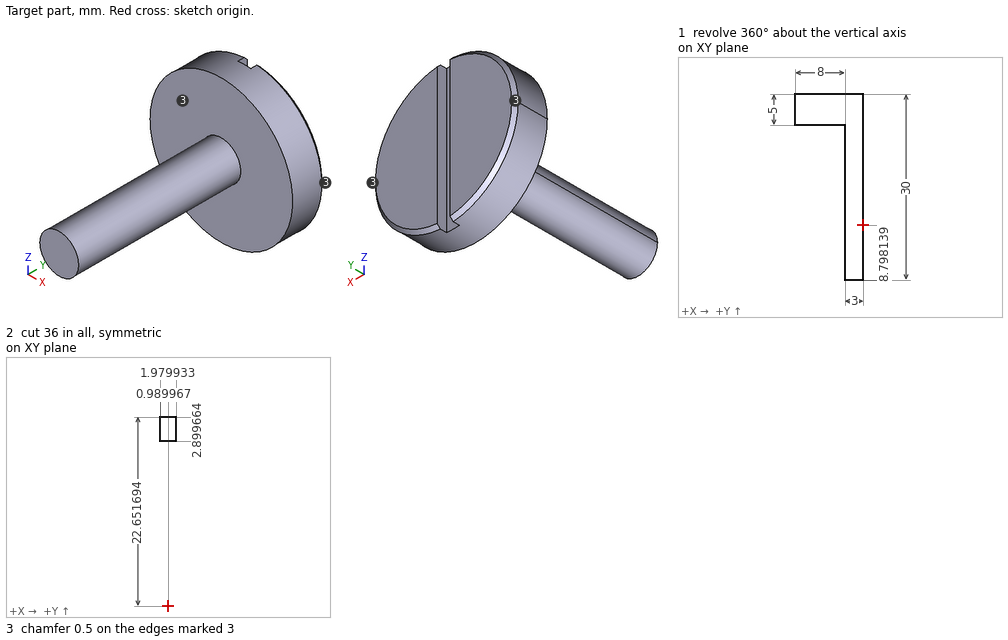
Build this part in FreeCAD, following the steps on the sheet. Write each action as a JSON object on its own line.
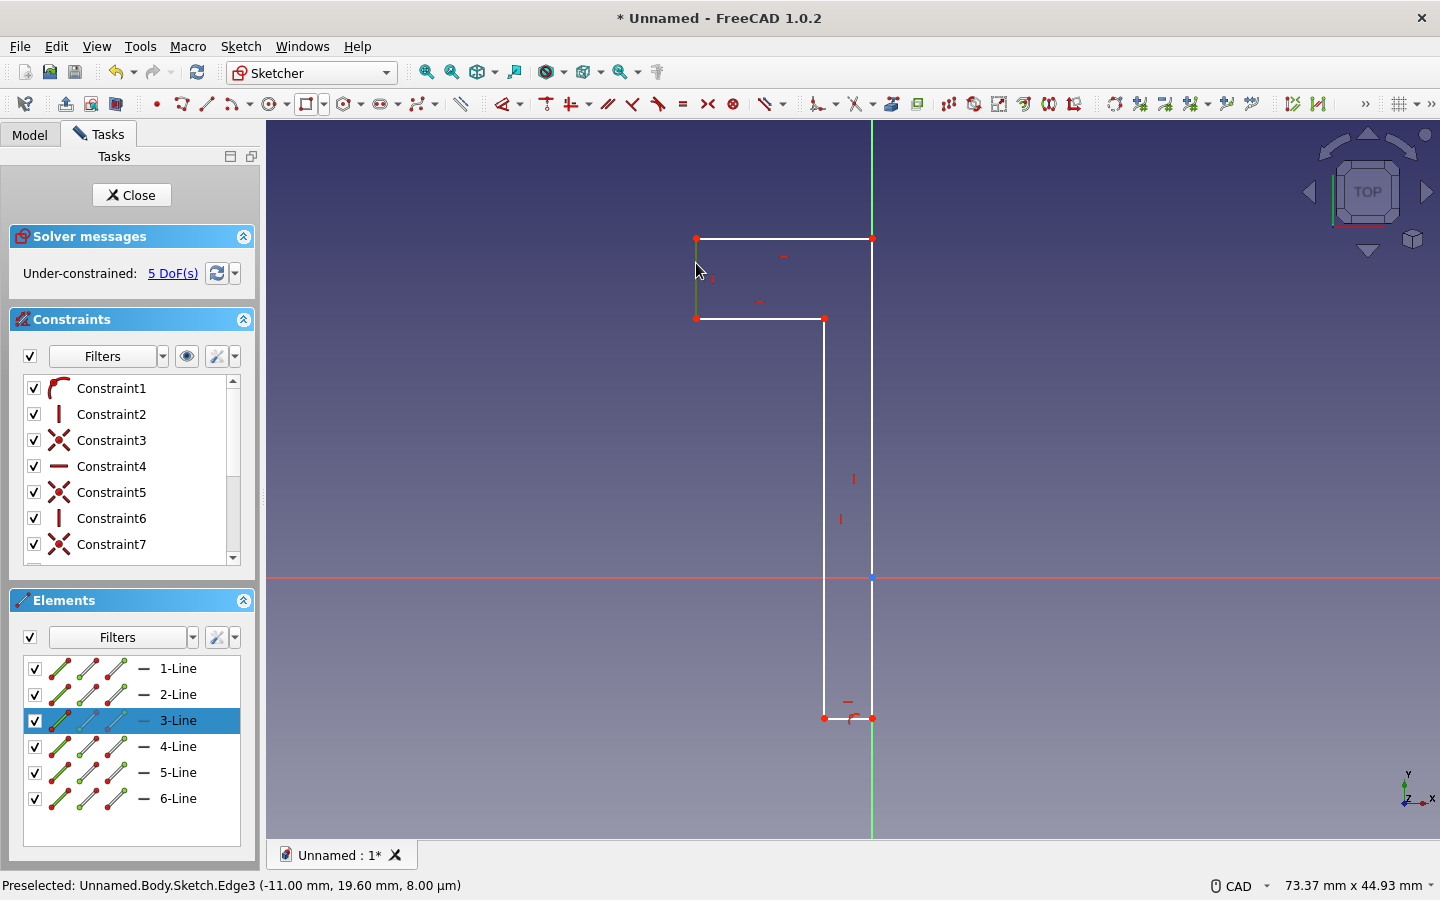
{"action": "left_click", "coordinate": [520, 104]}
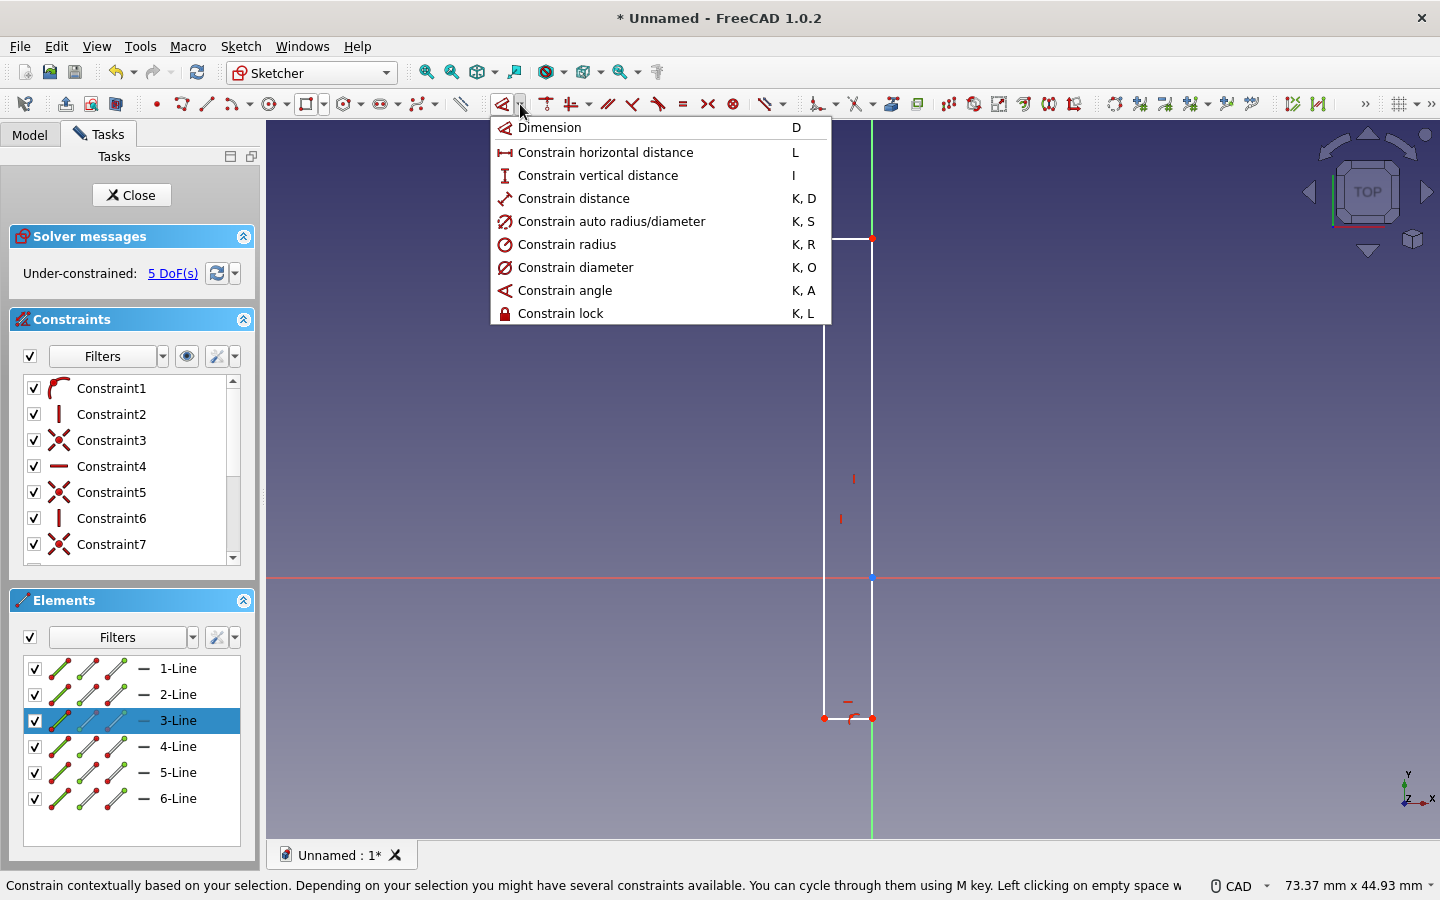
{"action": "left_click", "coordinate": [661, 176]}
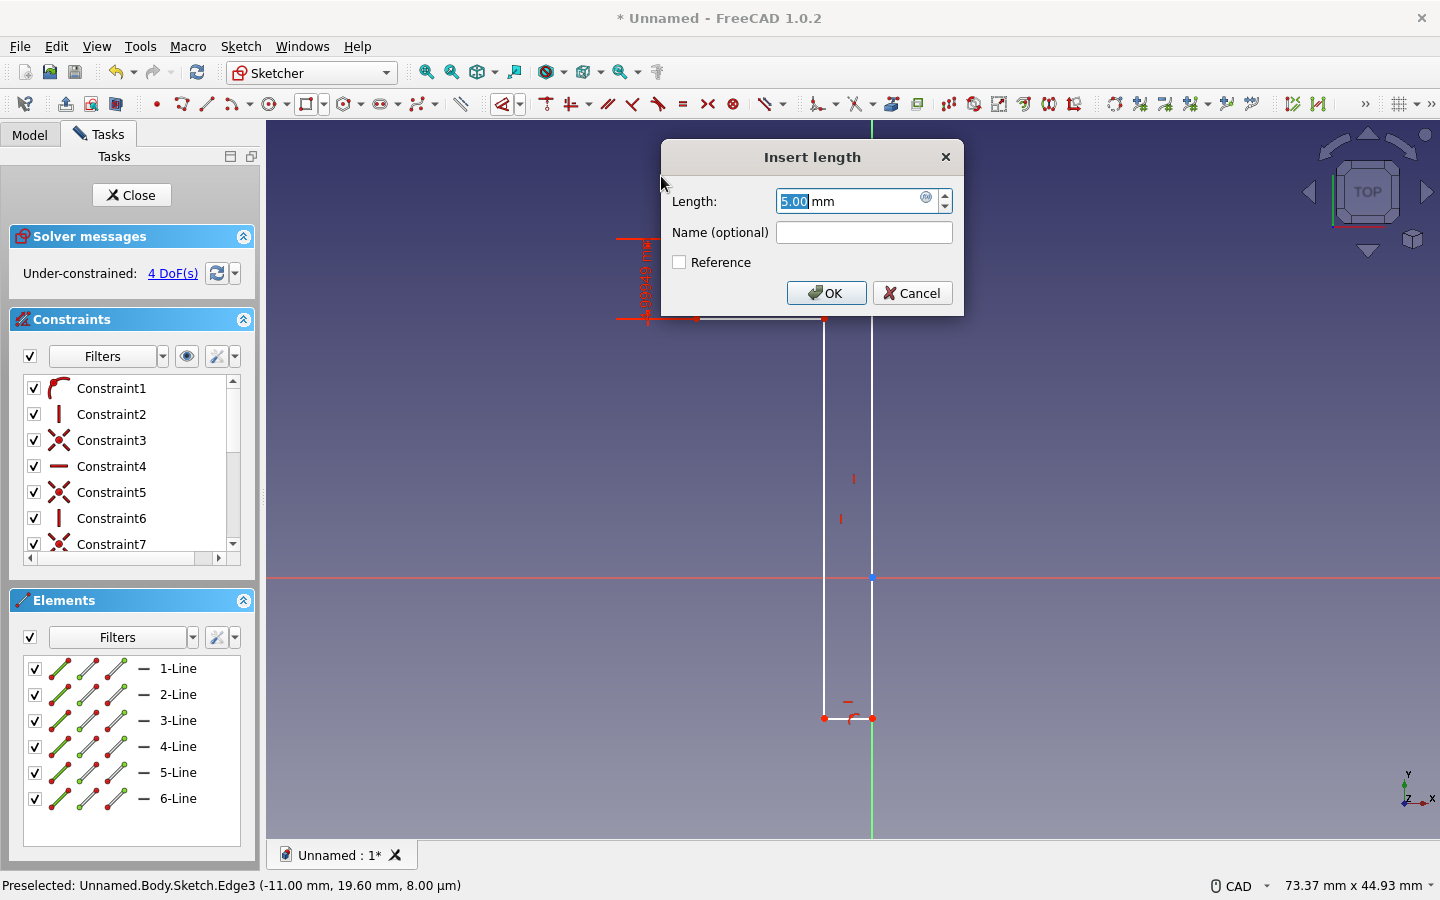
{"action": "type", "text": "5"}
{"action": "key", "text": "Return"}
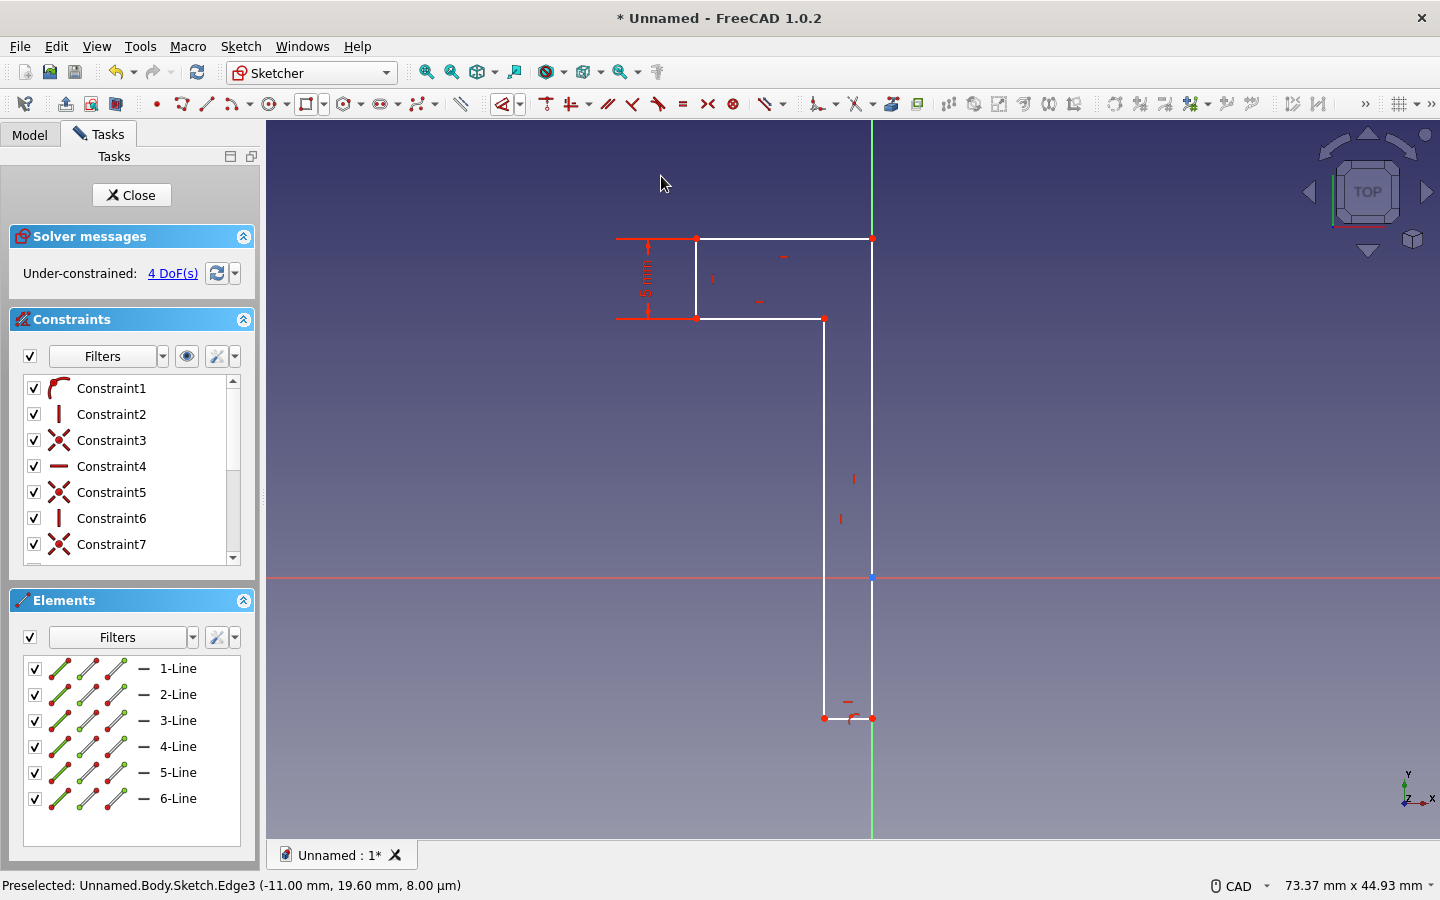
{"action": "left_click", "coordinate": [734, 319]}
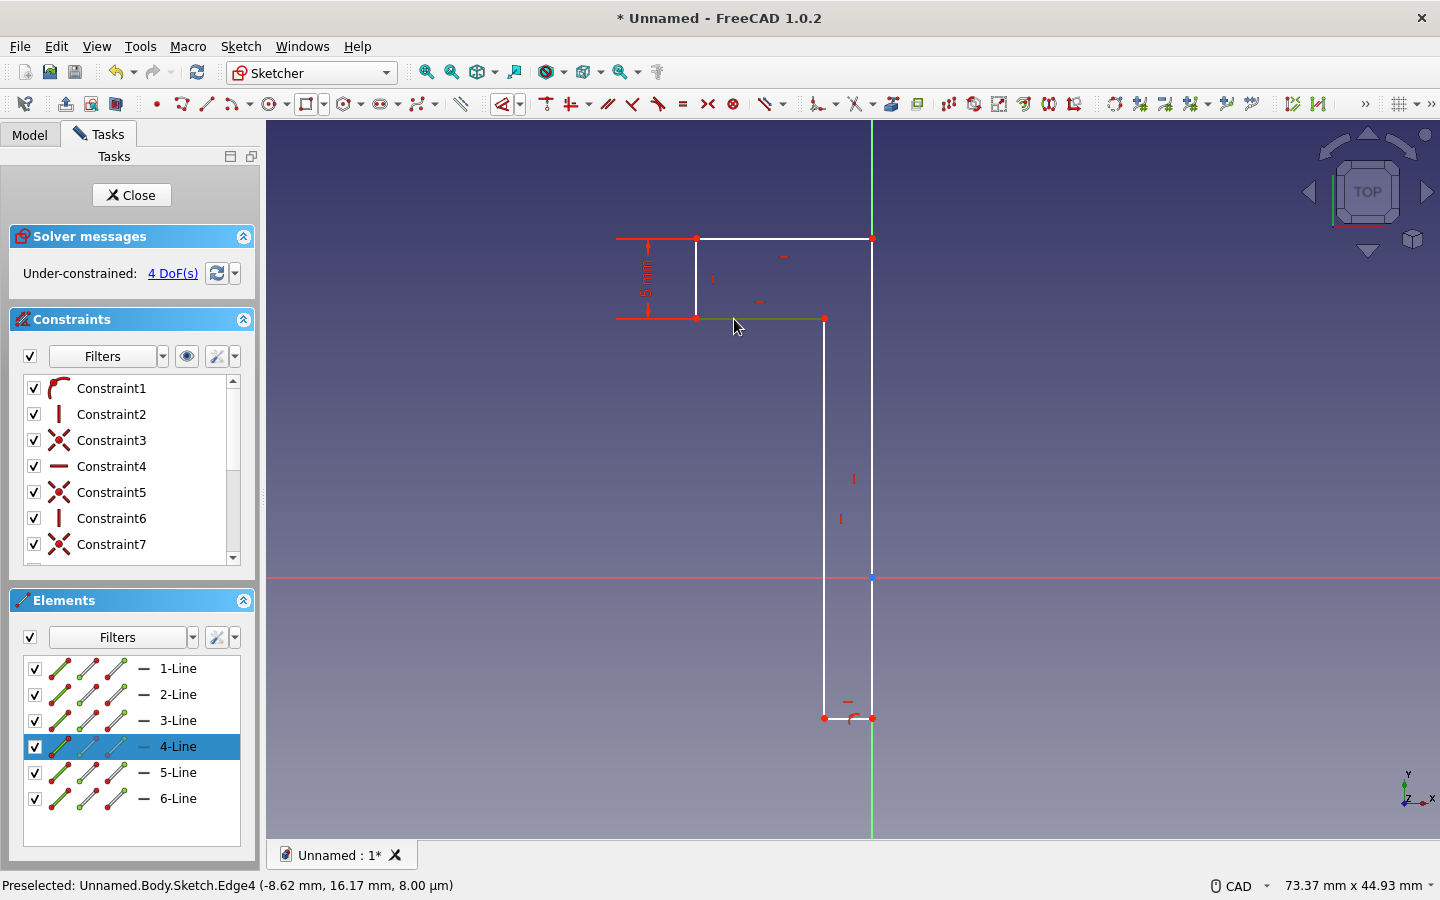
{"action": "key", "text": "l"}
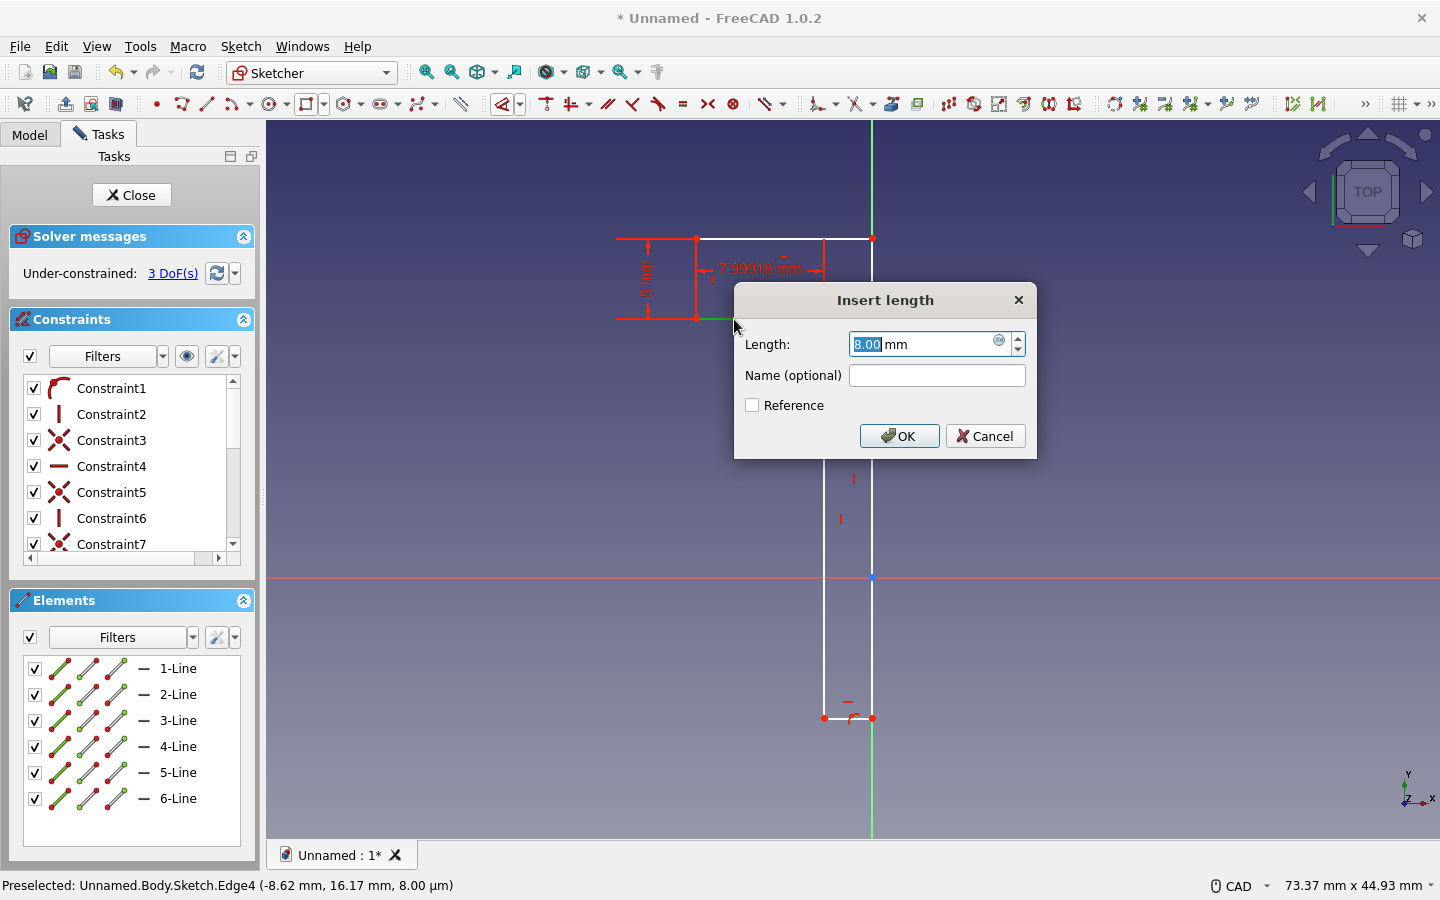
{"action": "type", "text": "8"}
{"action": "key", "text": "Return"}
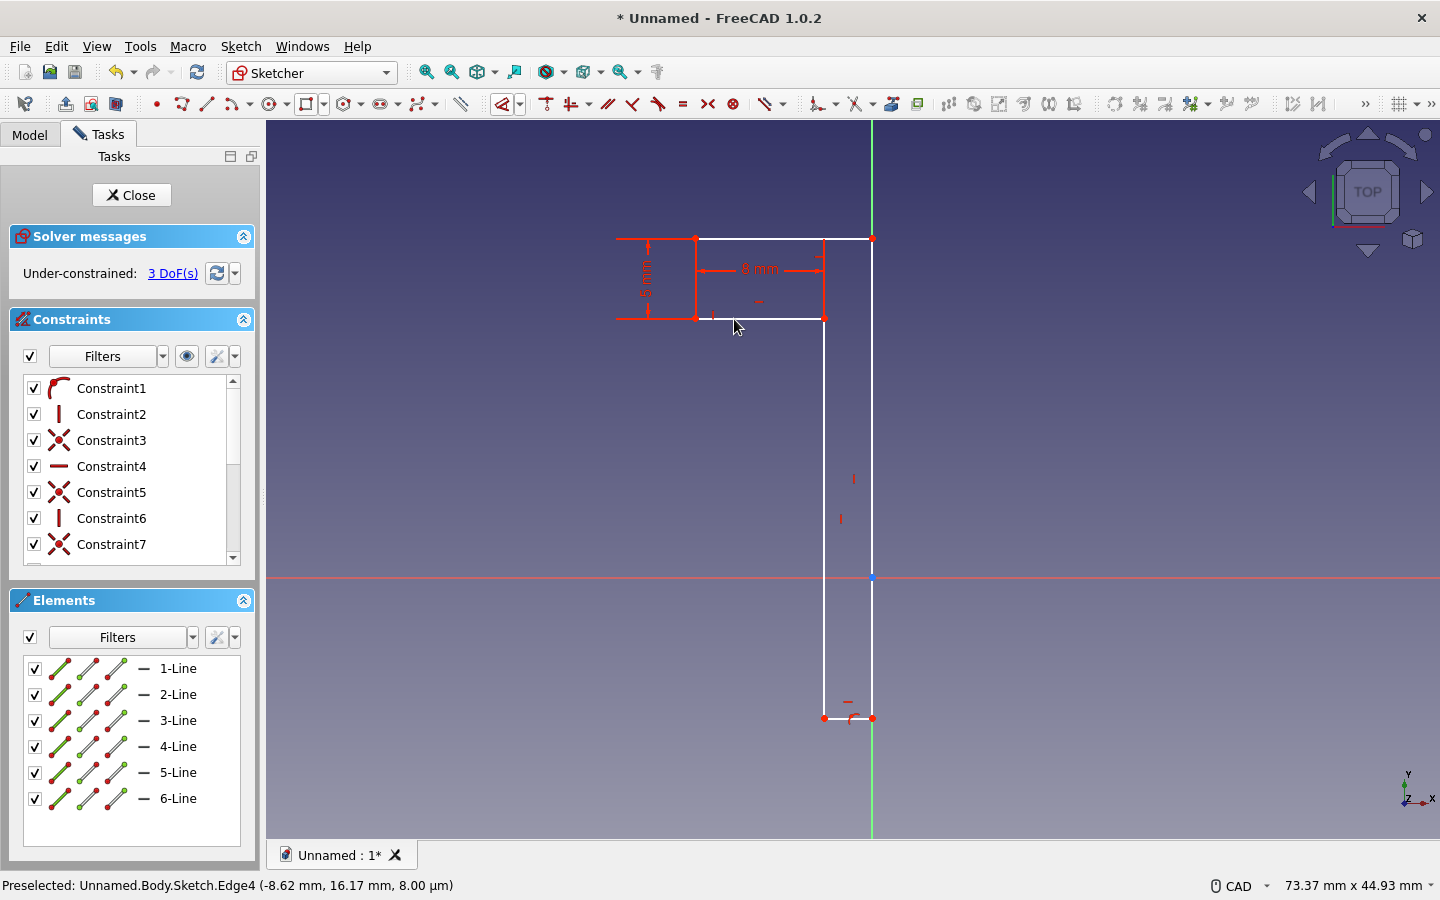
{"action": "left_click", "coordinate": [838, 719]}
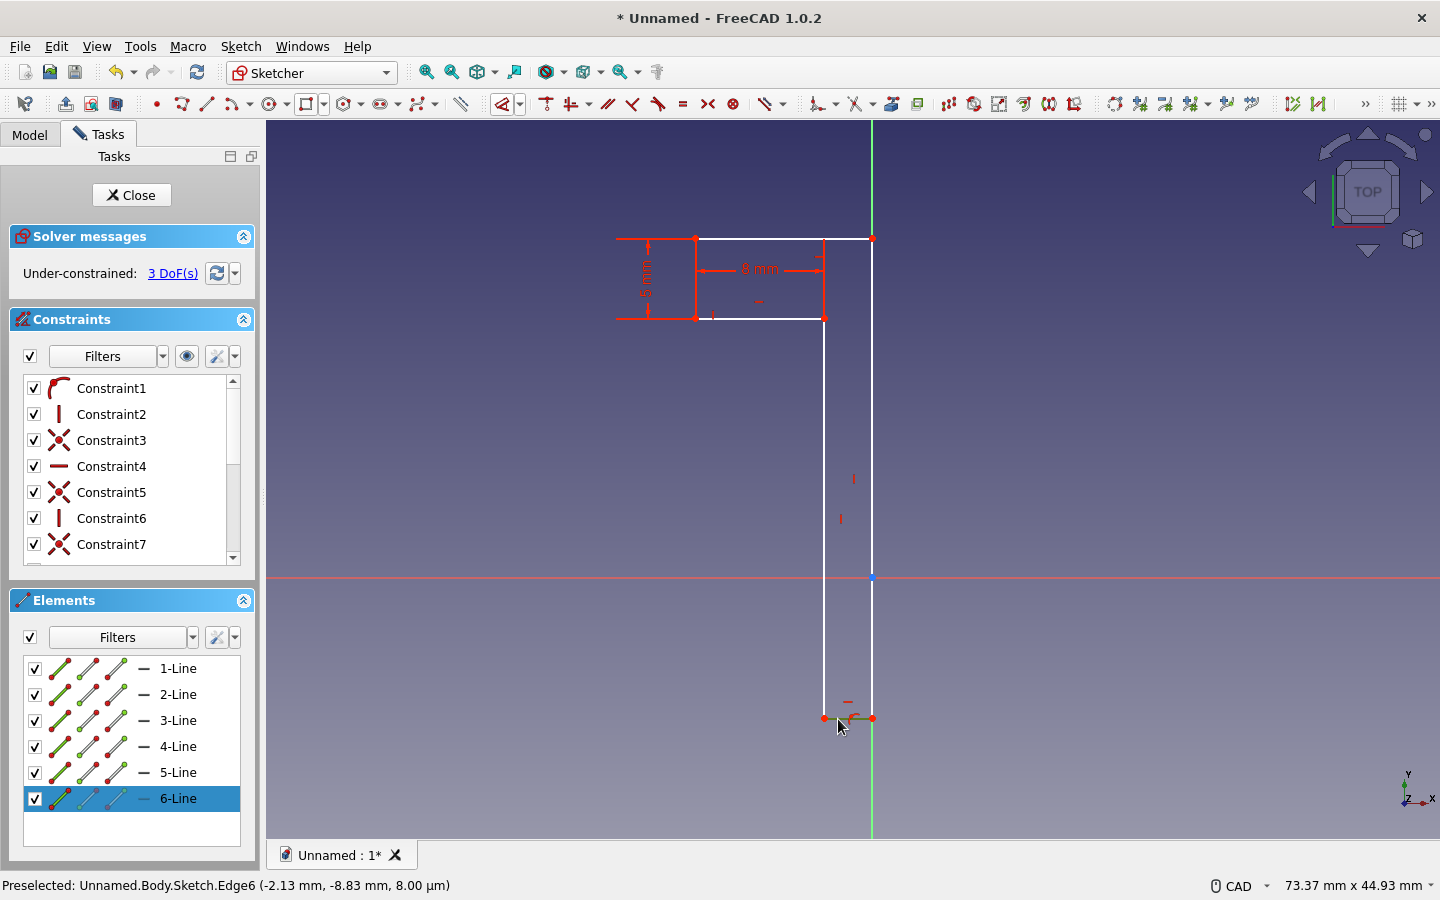
{"action": "key", "text": "l"}